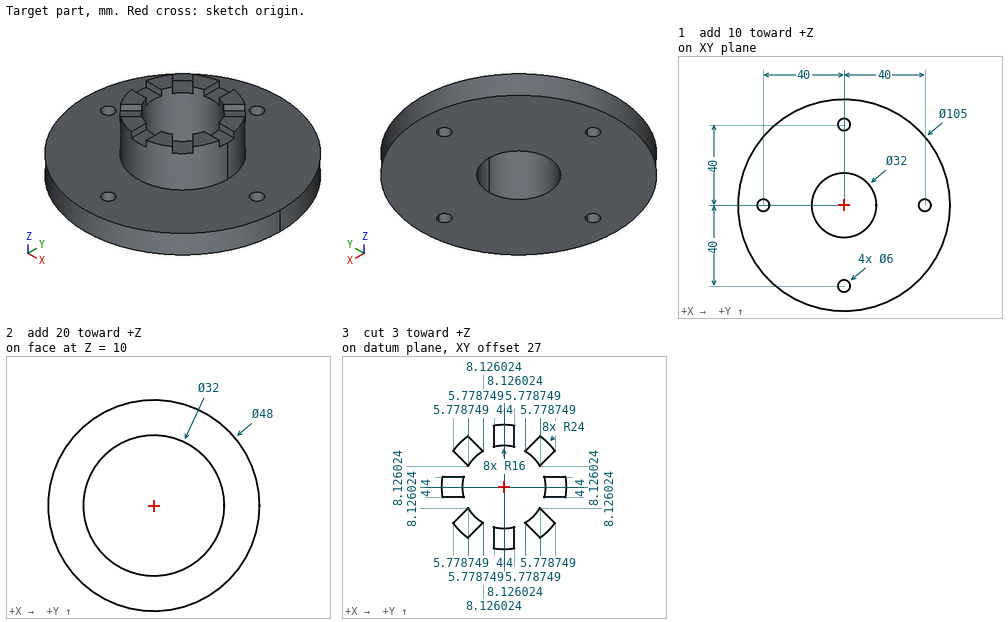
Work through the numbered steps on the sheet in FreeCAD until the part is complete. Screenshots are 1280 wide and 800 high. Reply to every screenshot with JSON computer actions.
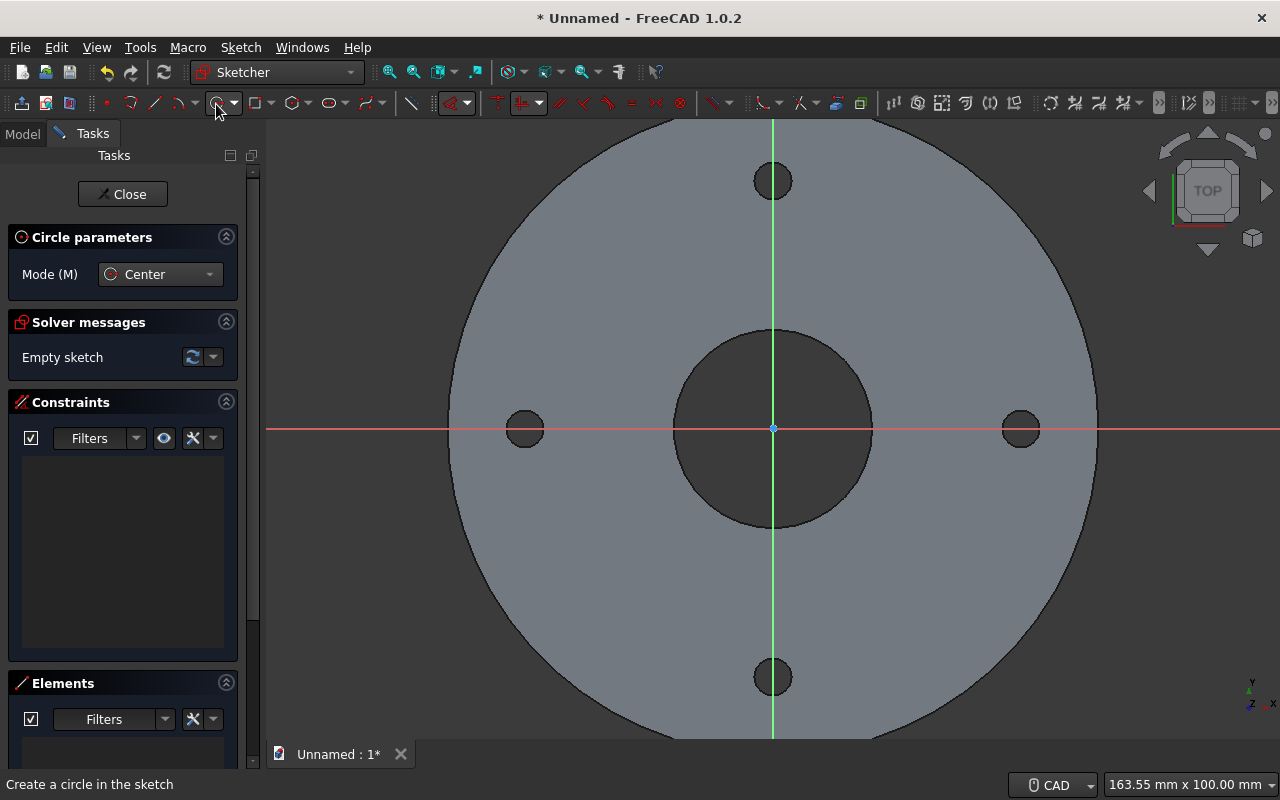
{"action": "left_click", "coordinate": [773, 429]}
{"action": "left_click", "coordinate": [878, 324]}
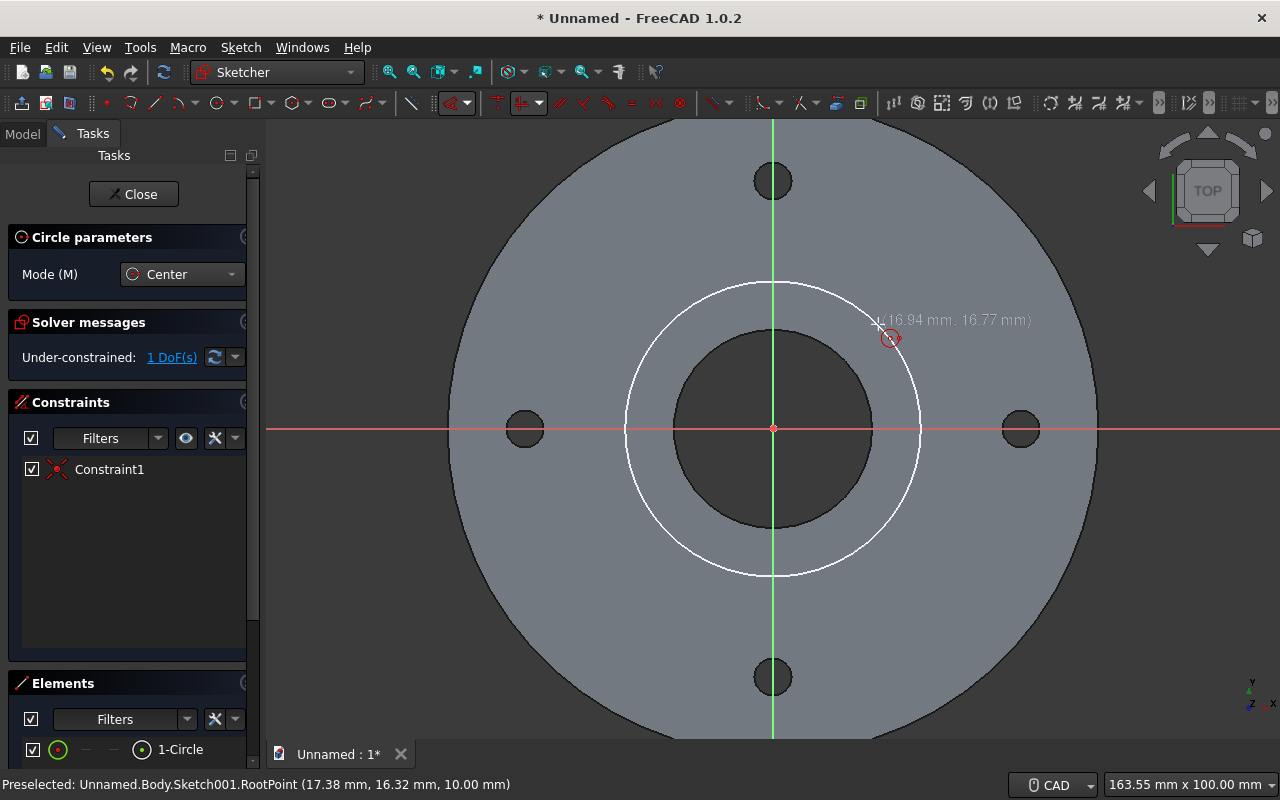
{"action": "left_click", "coordinate": [773, 429]}
{"action": "left_click", "coordinate": [843, 359]}
{"action": "key", "text": "Escape"}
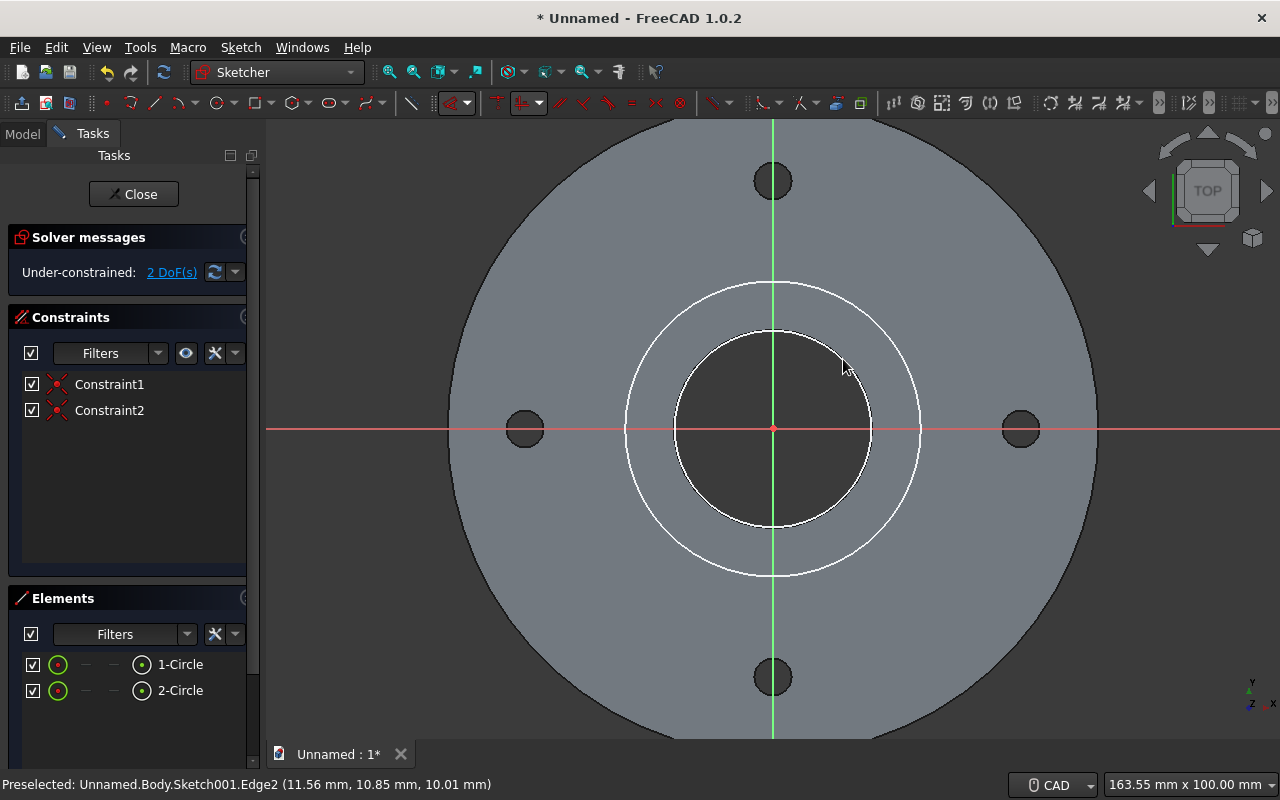
{"action": "left_click", "coordinate": [877, 324]}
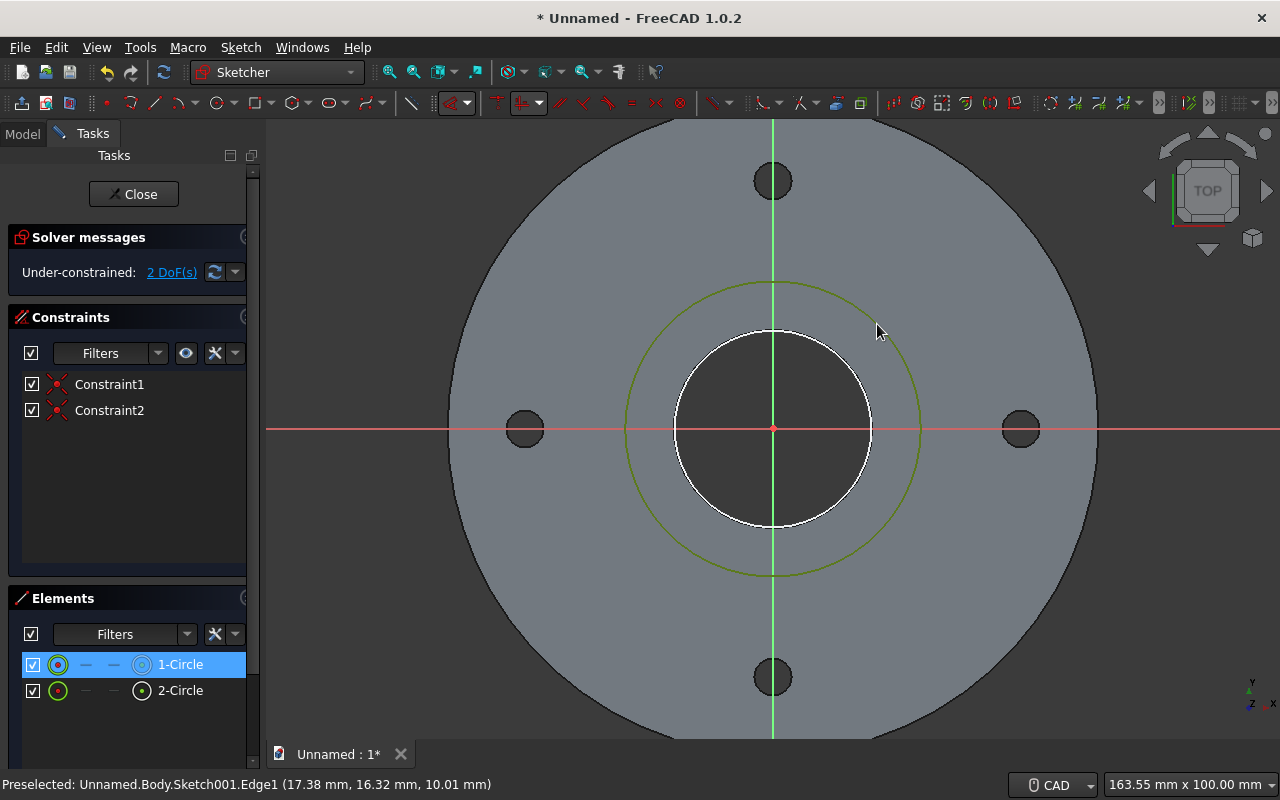
{"action": "key", "text": "k o"}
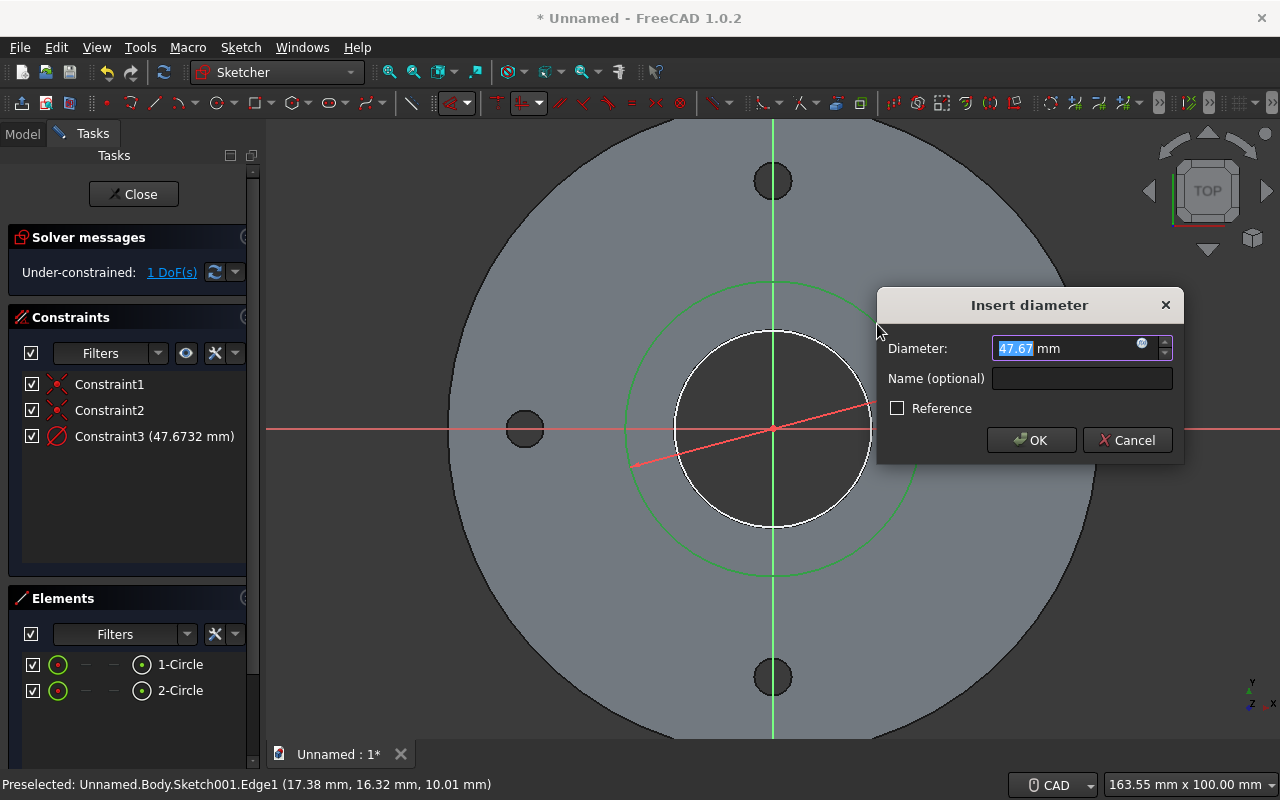
{"action": "type", "text": "48"}
{"action": "key", "text": "Return"}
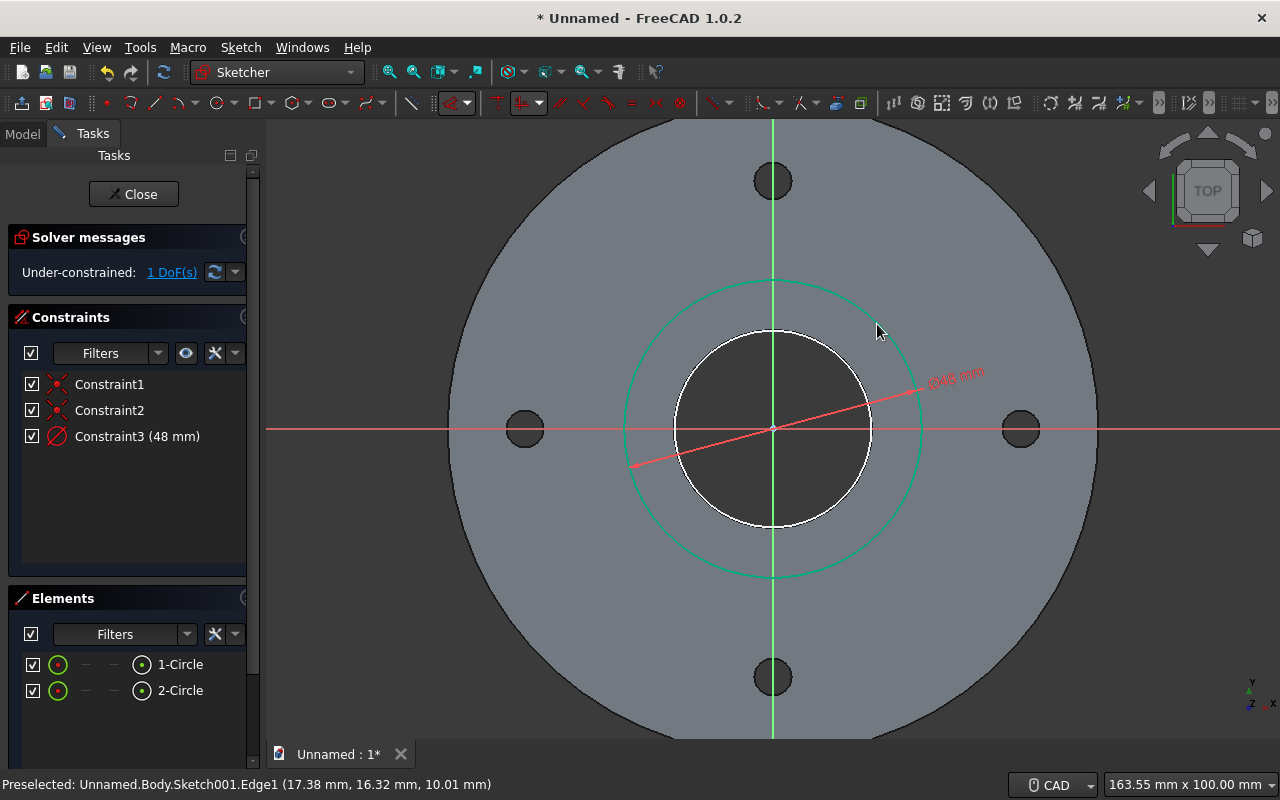
{"action": "left_click", "coordinate": [842, 359]}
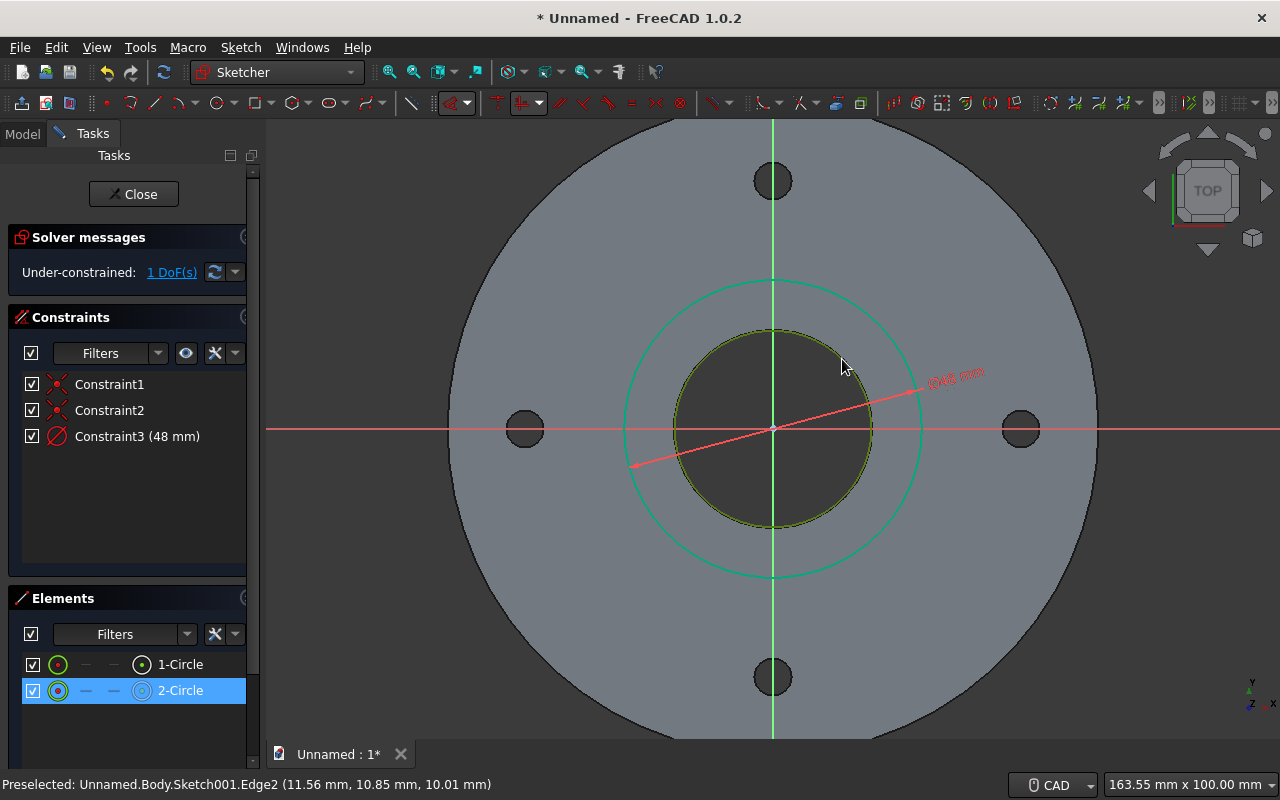
{"action": "left_click", "coordinate": [470, 104]}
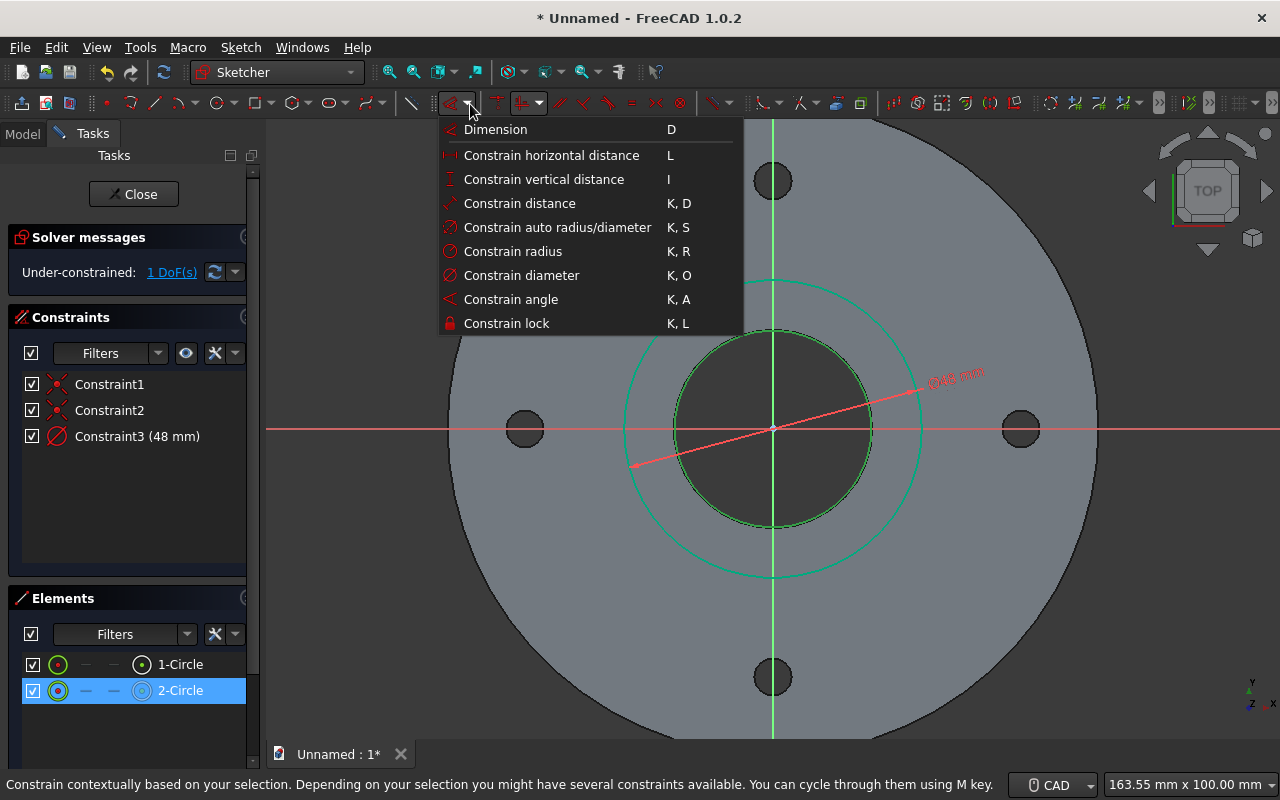
{"action": "left_click", "coordinate": [591, 275]}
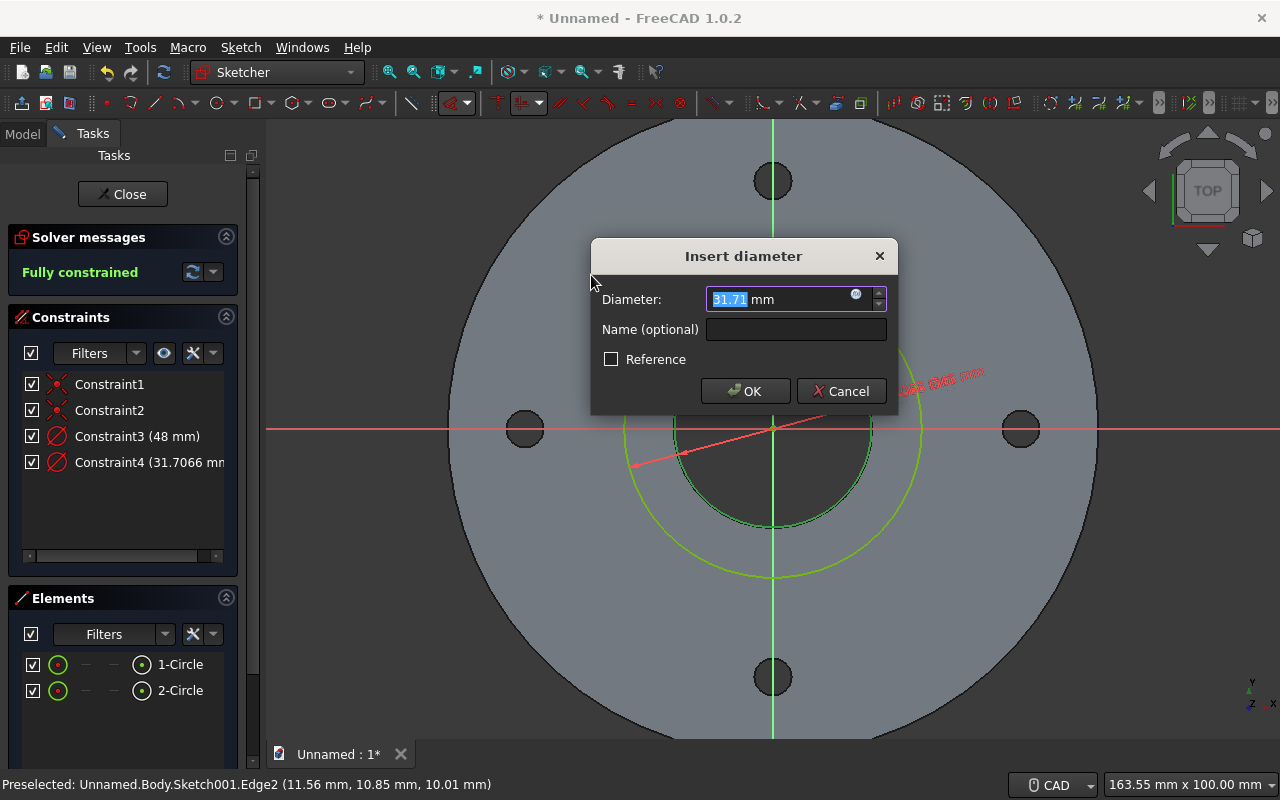
{"action": "type", "text": "32"}
{"action": "key", "text": "Return"}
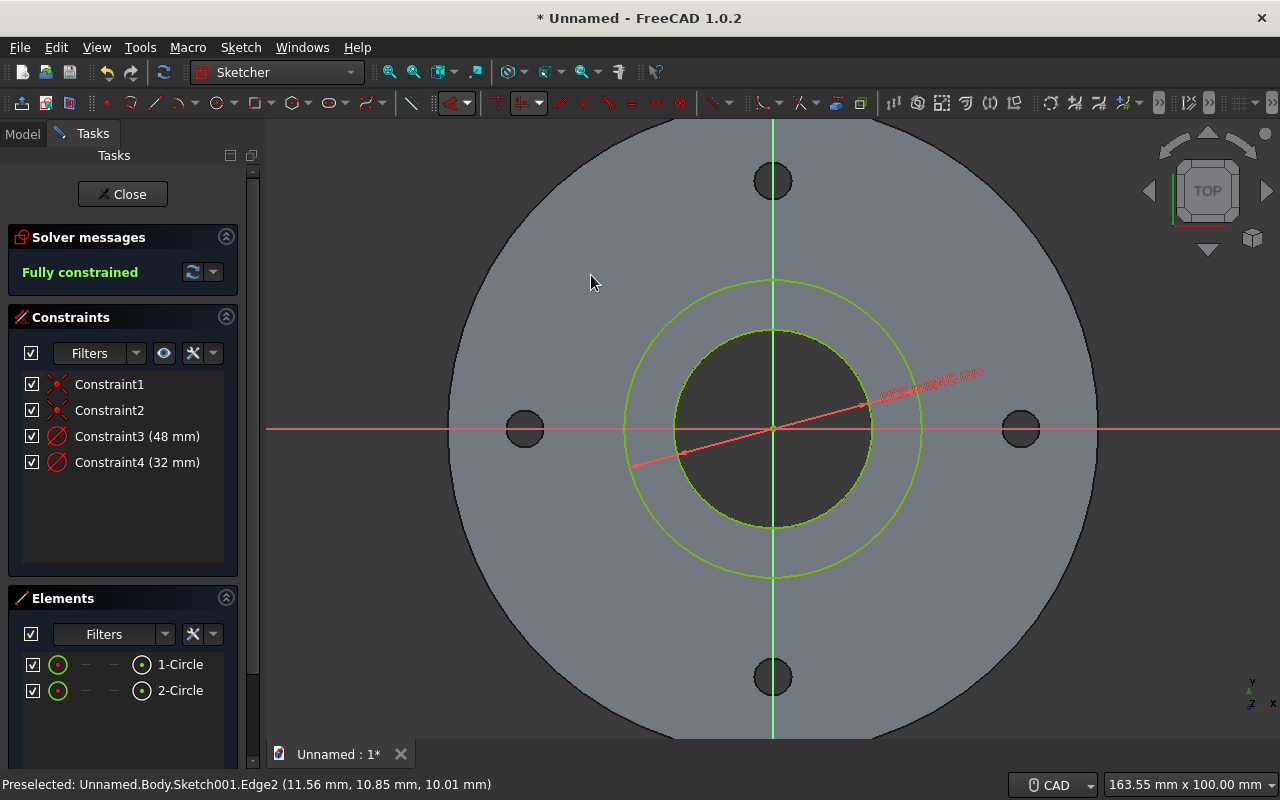
{"action": "left_click", "coordinate": [123, 194]}